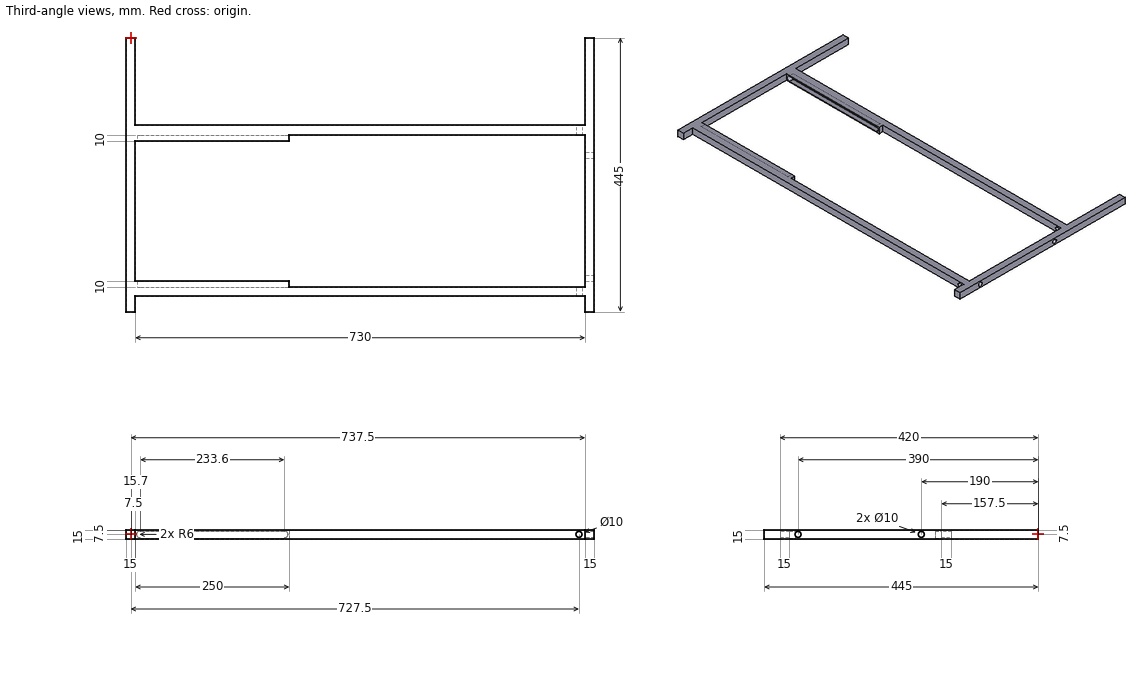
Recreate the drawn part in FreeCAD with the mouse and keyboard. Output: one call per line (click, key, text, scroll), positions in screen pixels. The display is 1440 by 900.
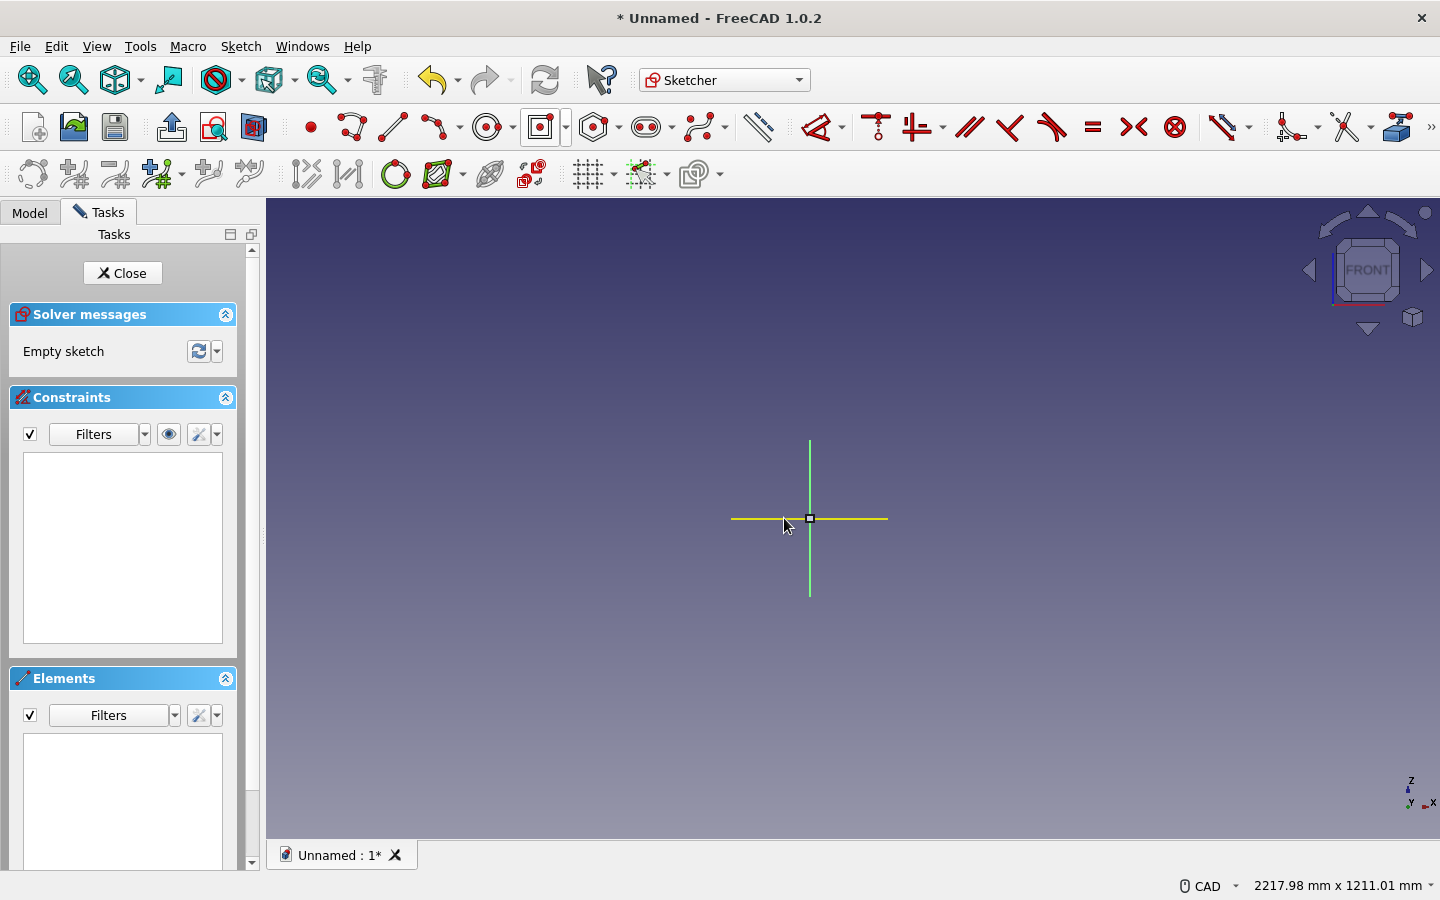
scroll(1226, 518, up, 15)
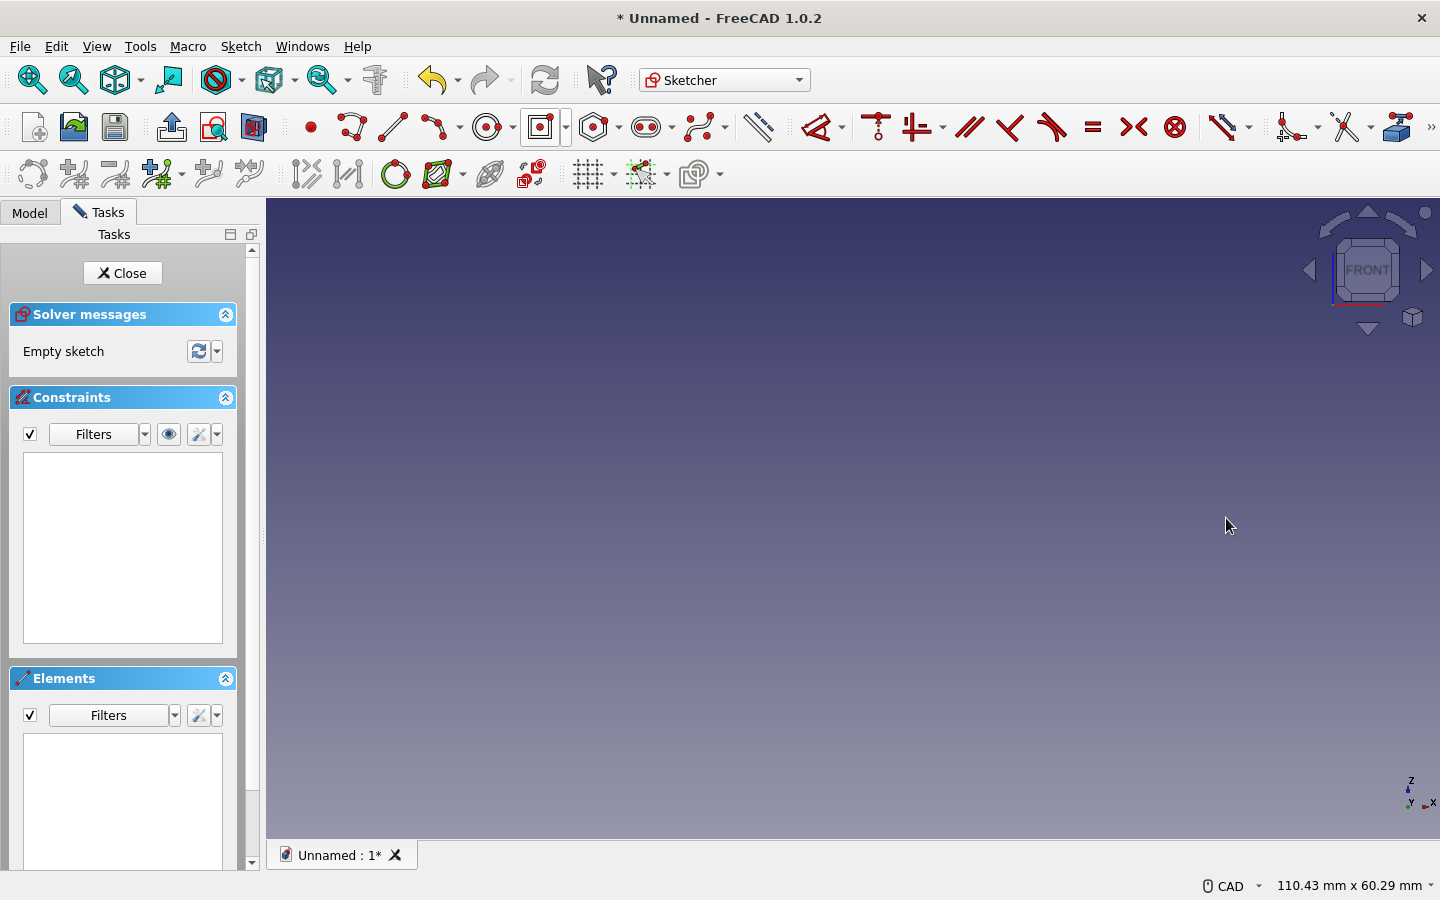
scroll(759, 518, up, 5)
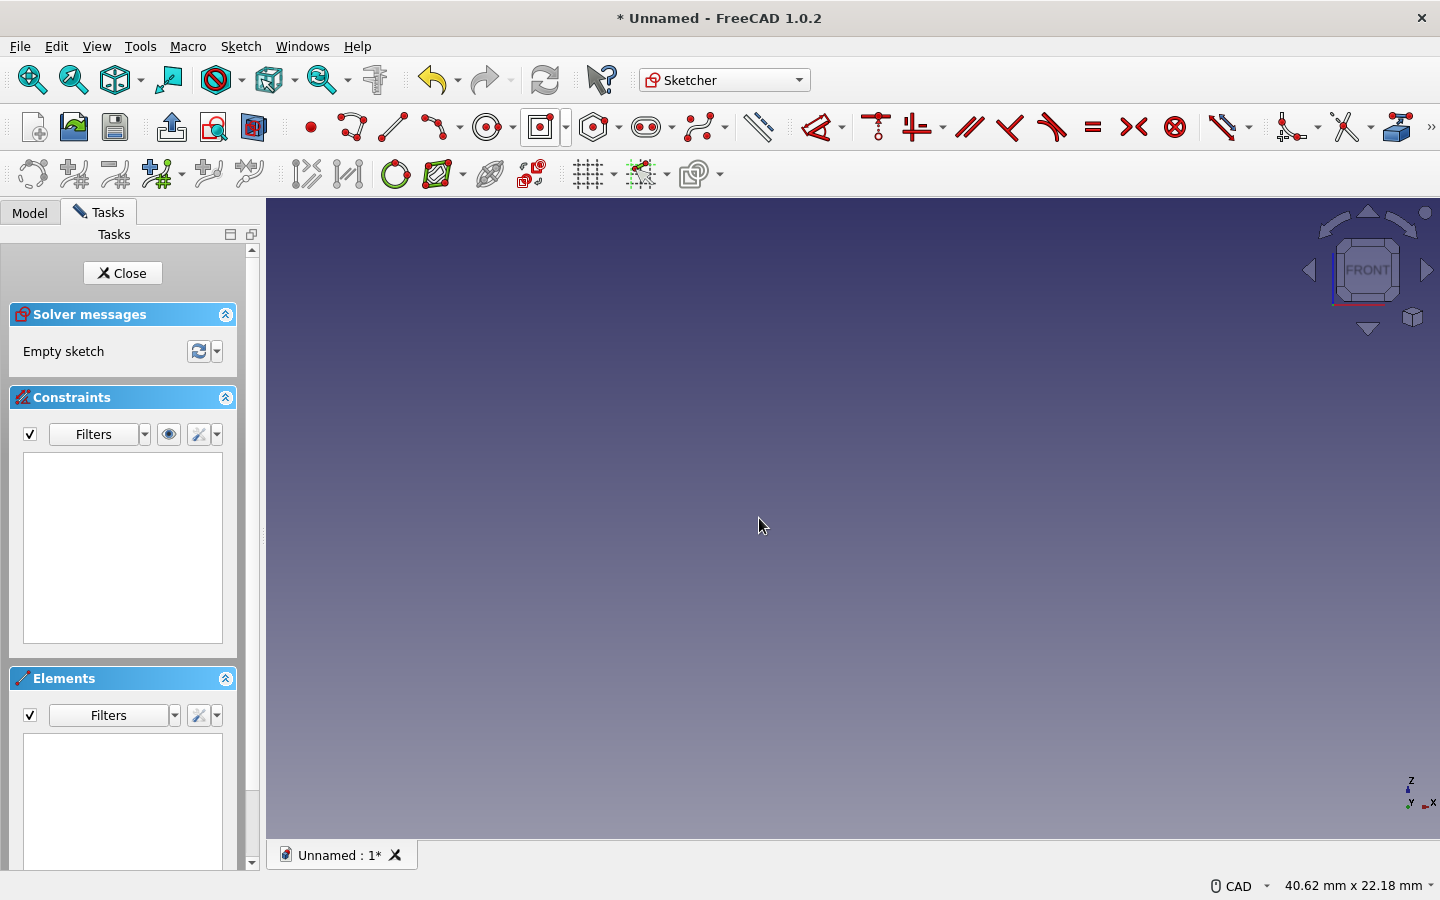
click(566, 128)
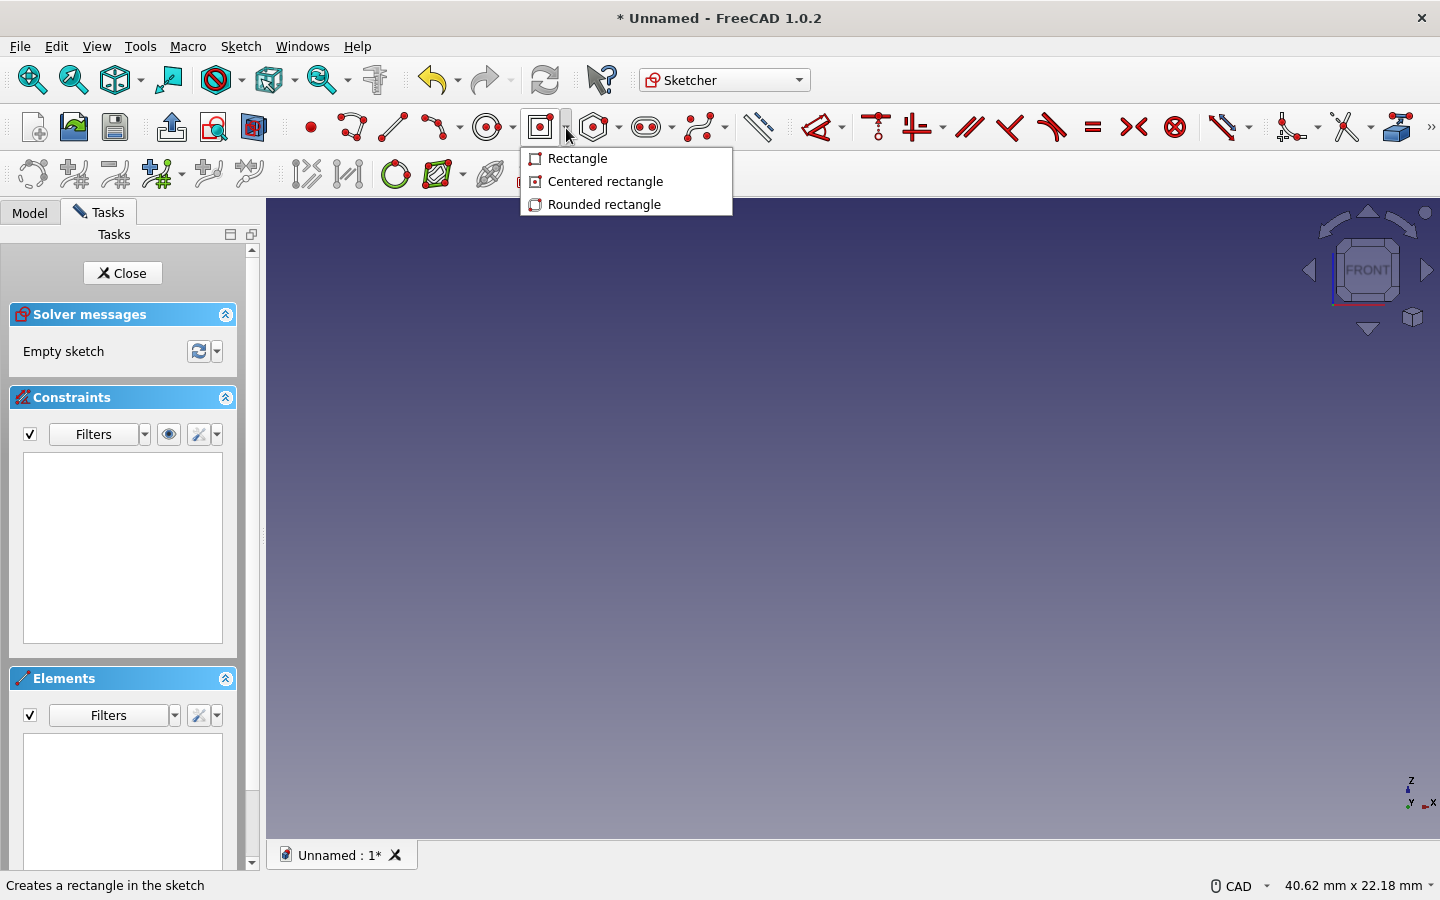
click(626, 158)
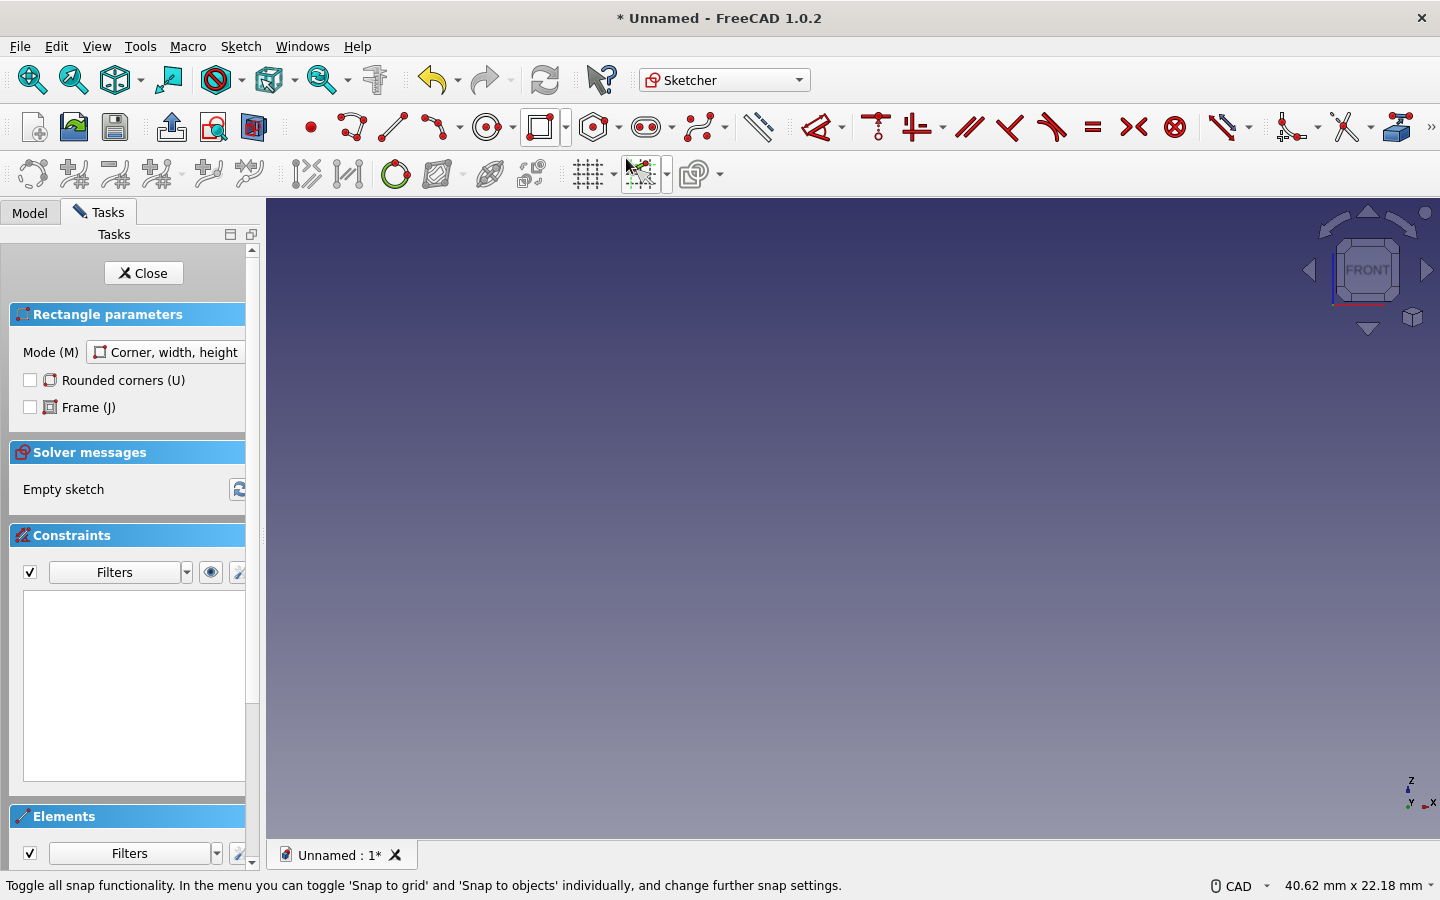
click(567, 302)
click(1001, 735)
key(Escape)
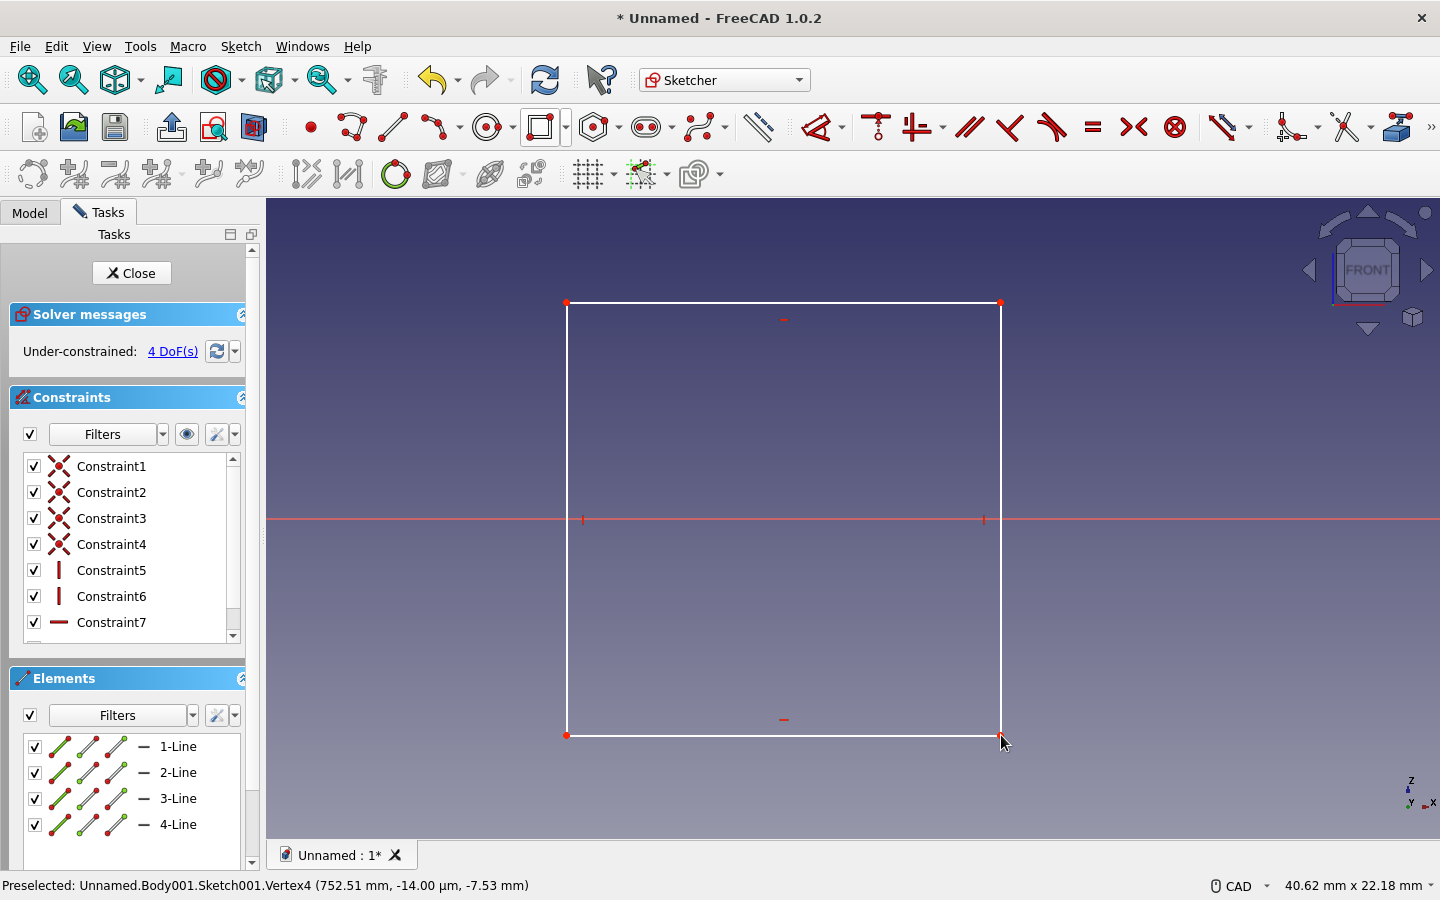
click(816, 128)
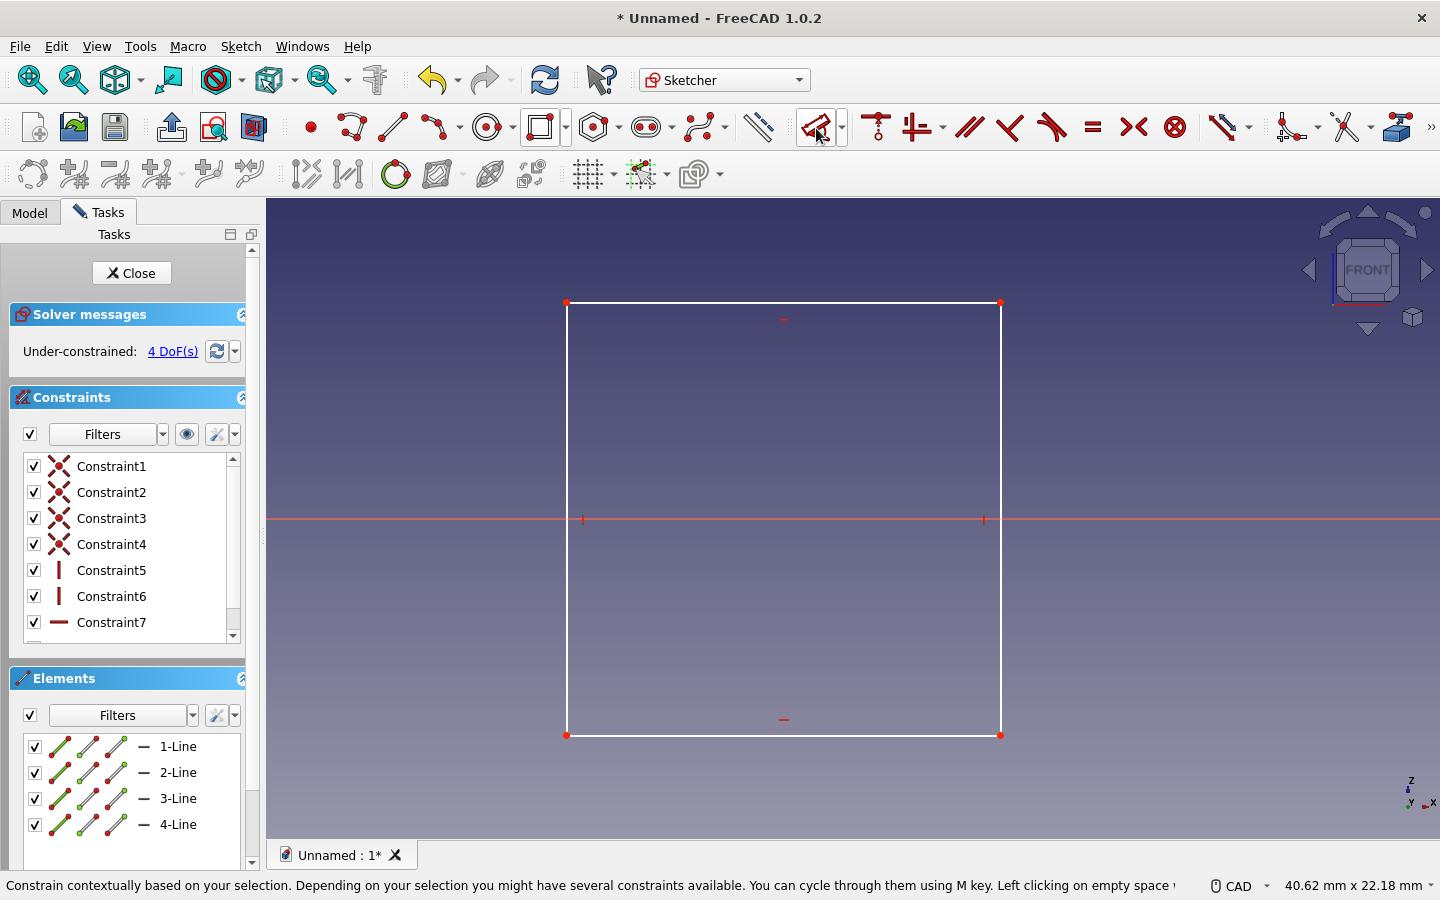
click(567, 433)
click(533, 420)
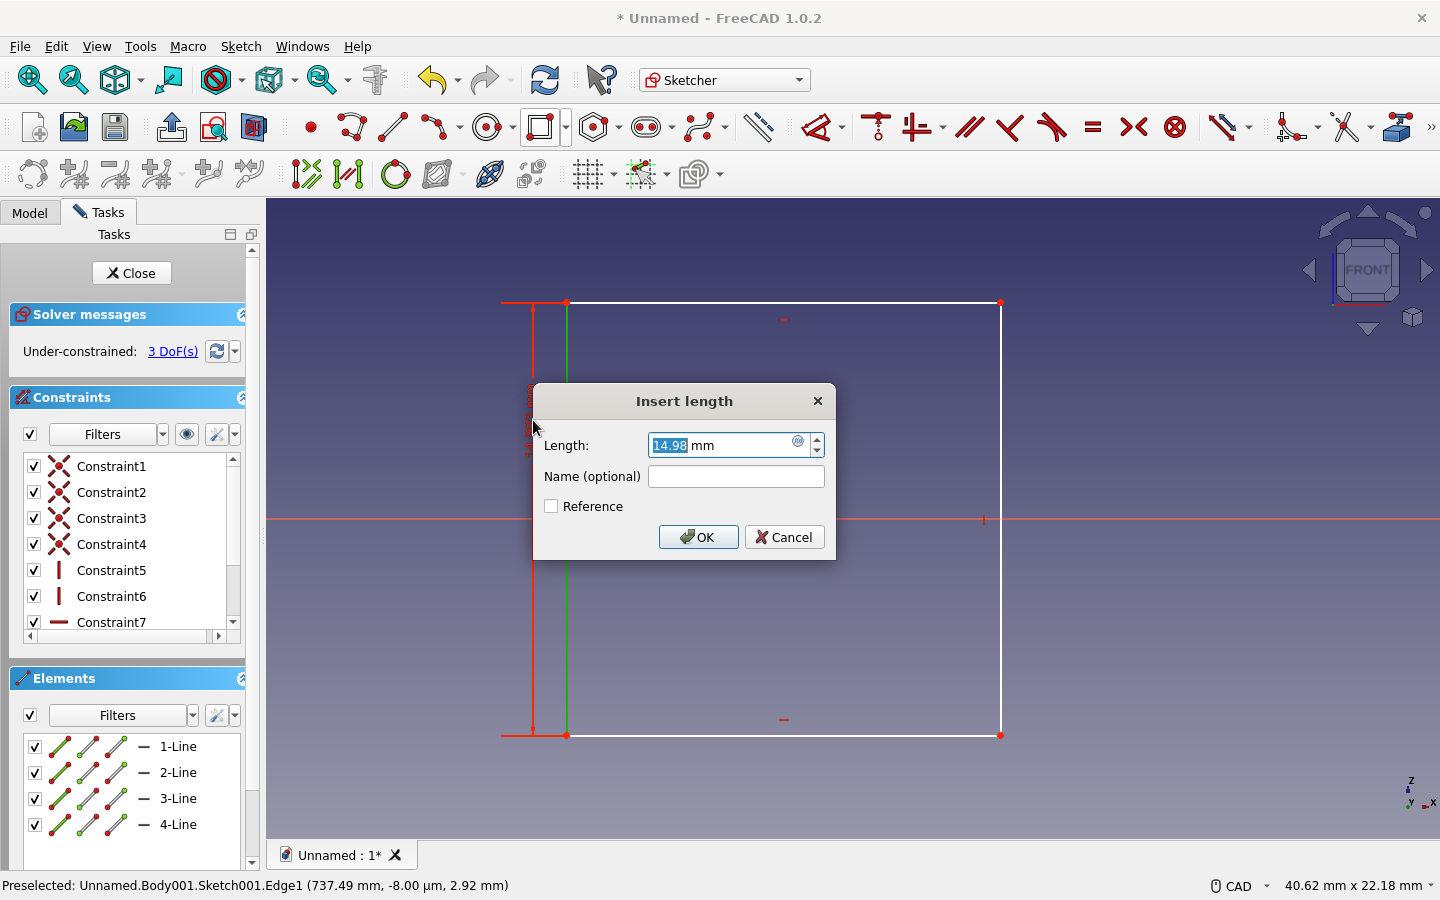
text(15)
key(Return)